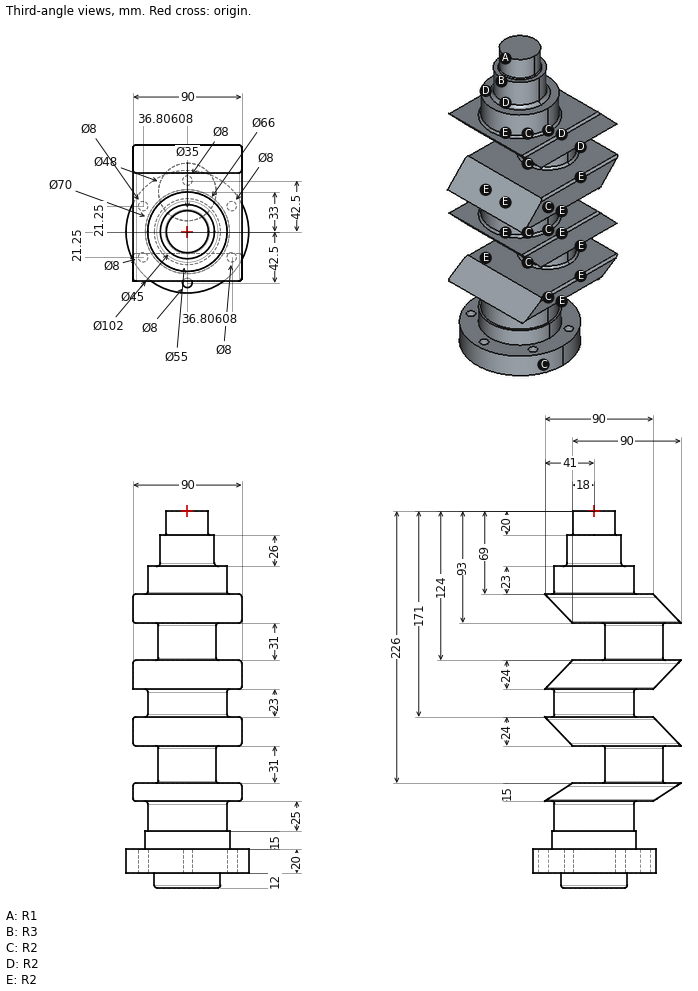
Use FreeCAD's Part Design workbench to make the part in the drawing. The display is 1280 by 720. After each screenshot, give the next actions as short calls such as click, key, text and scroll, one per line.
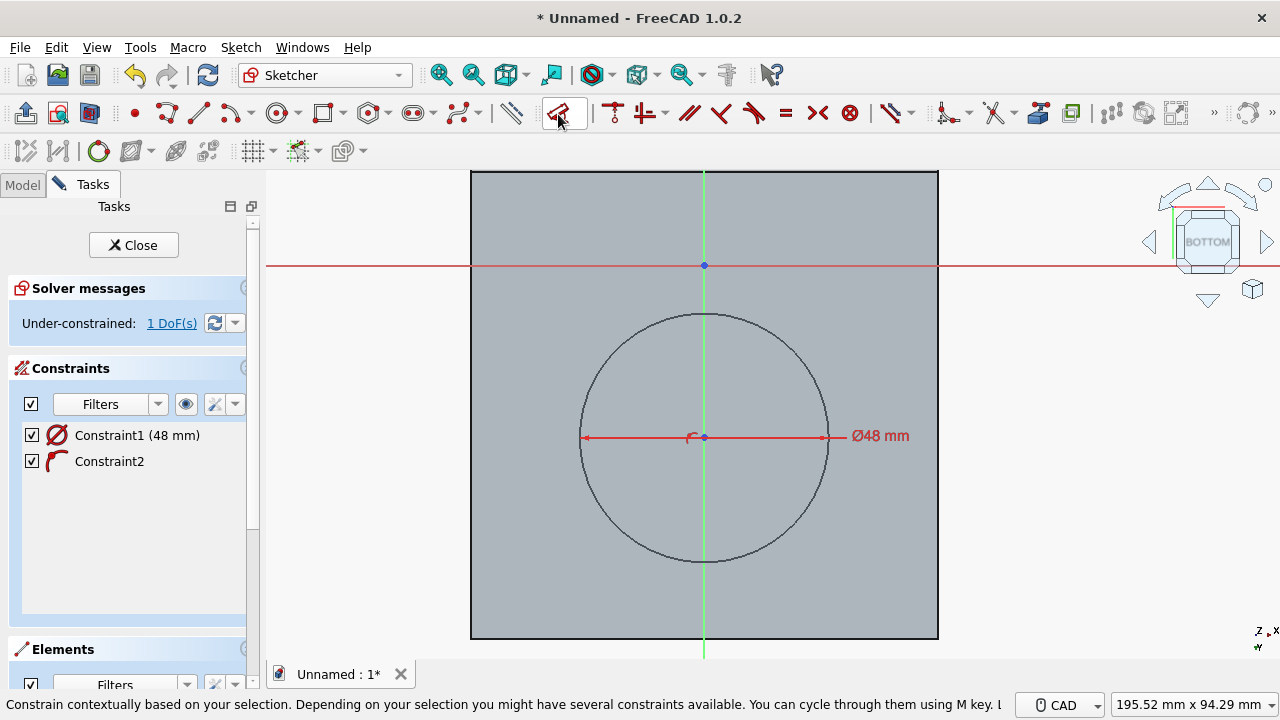
click(704, 438)
click(738, 352)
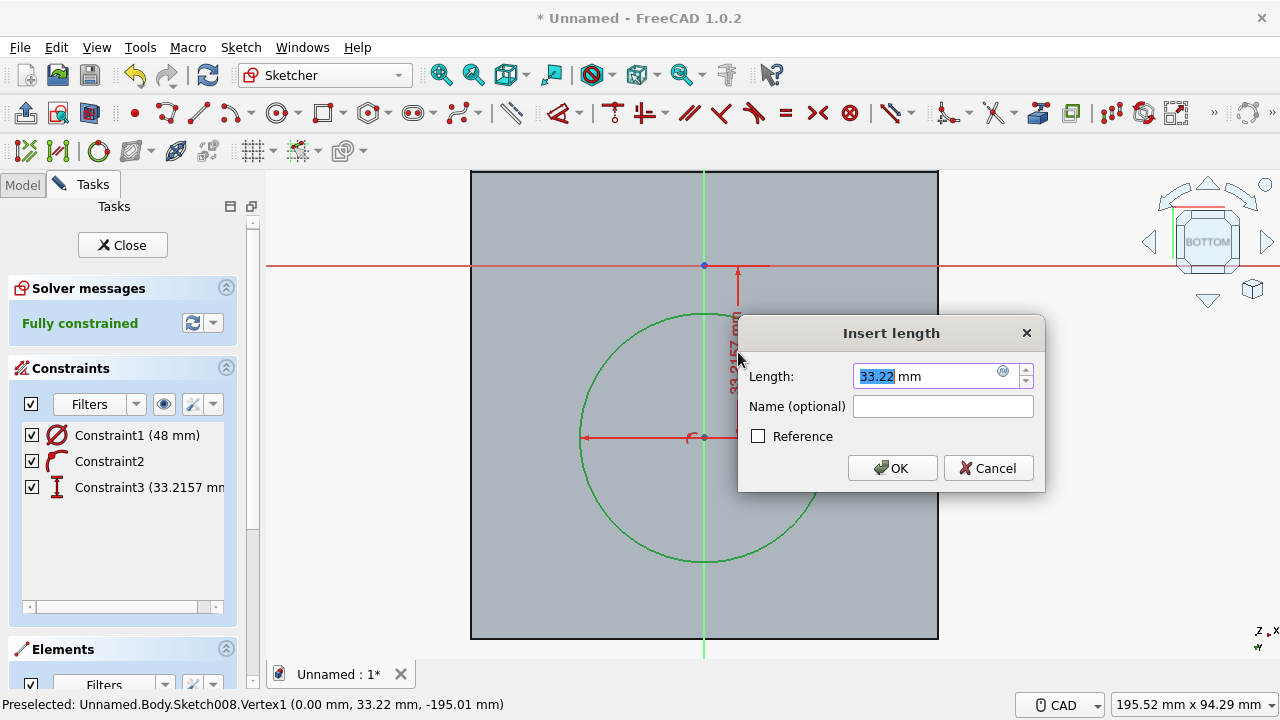
text(33)
key(Return)
key(Escape)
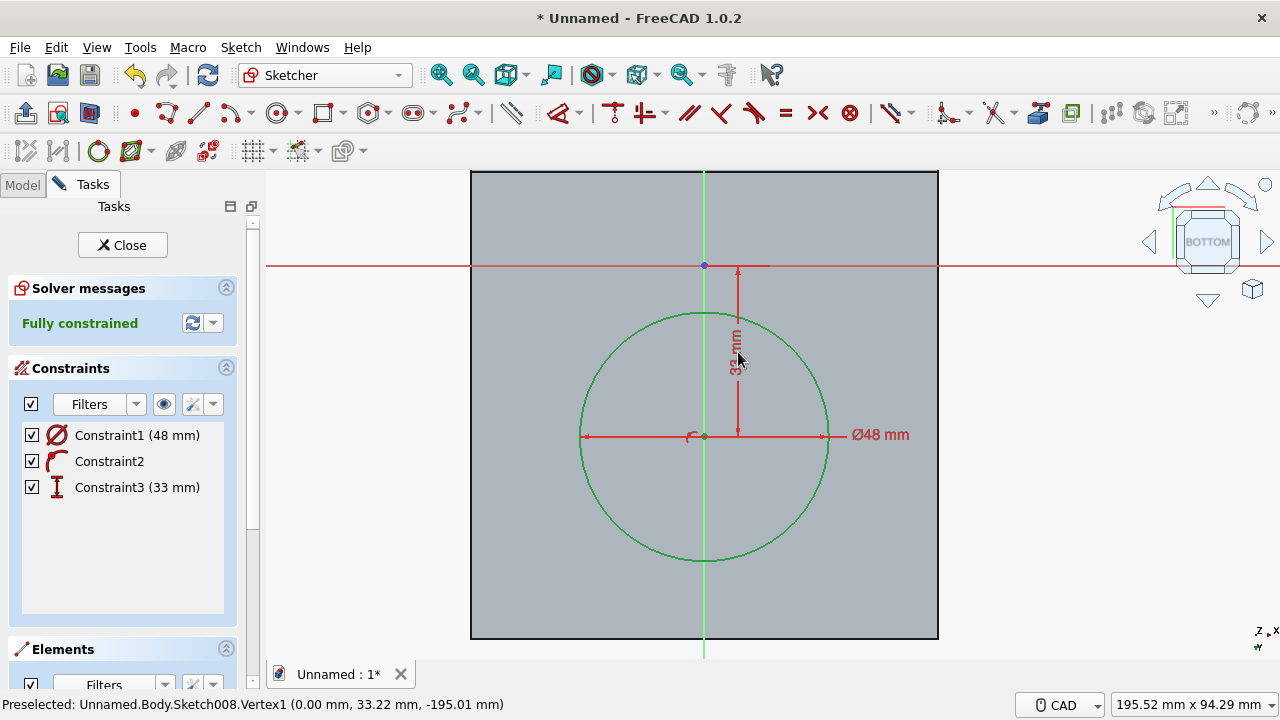
click(123, 245)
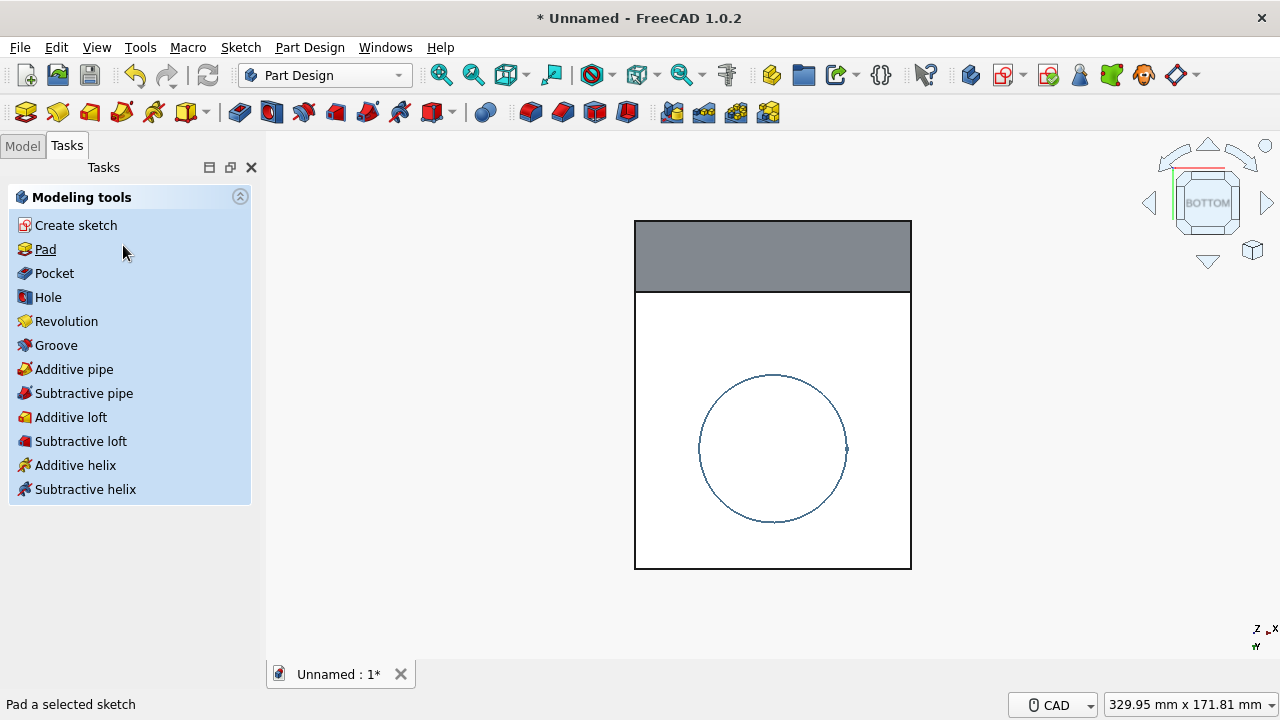
click(26, 112)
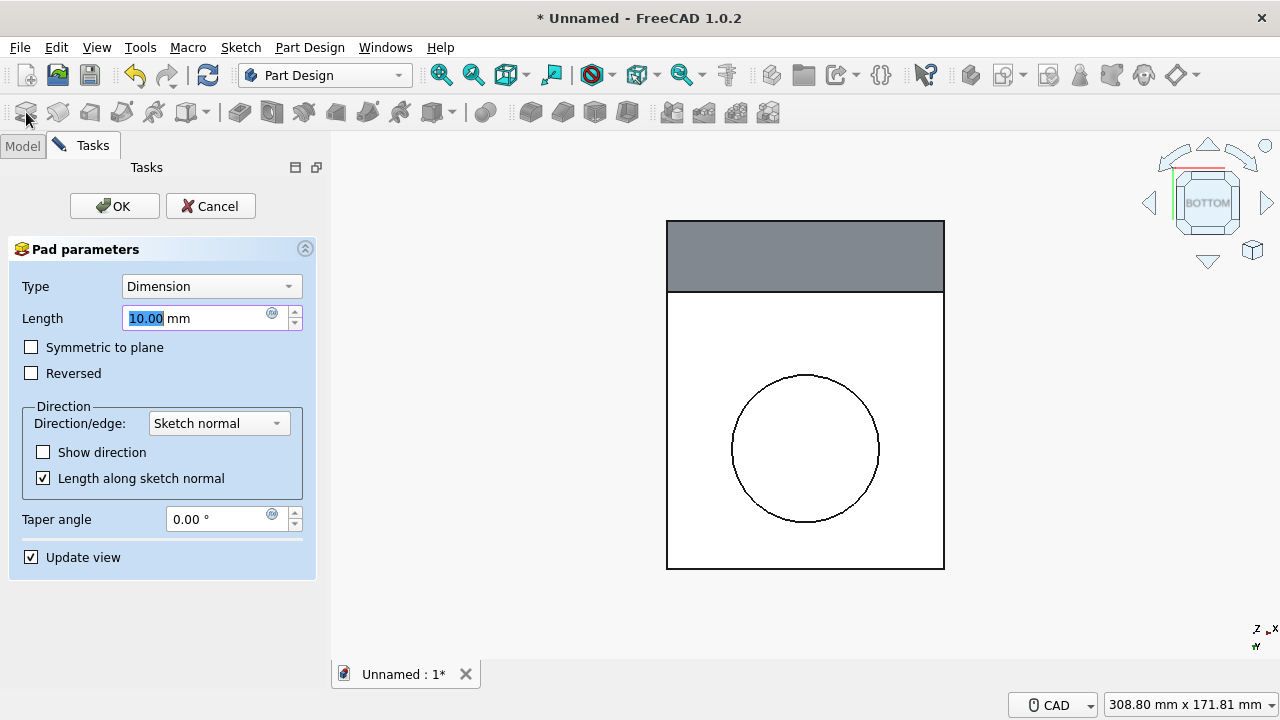
text(31)
key(Tab)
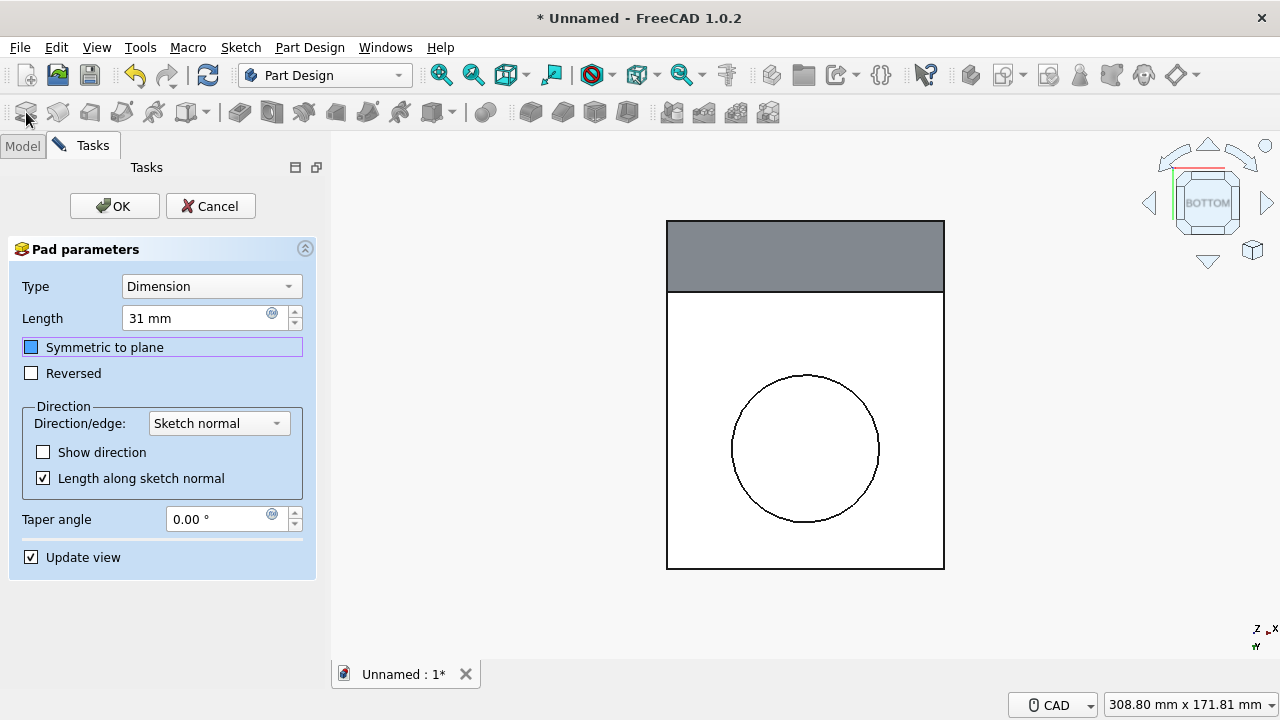
click(115, 206)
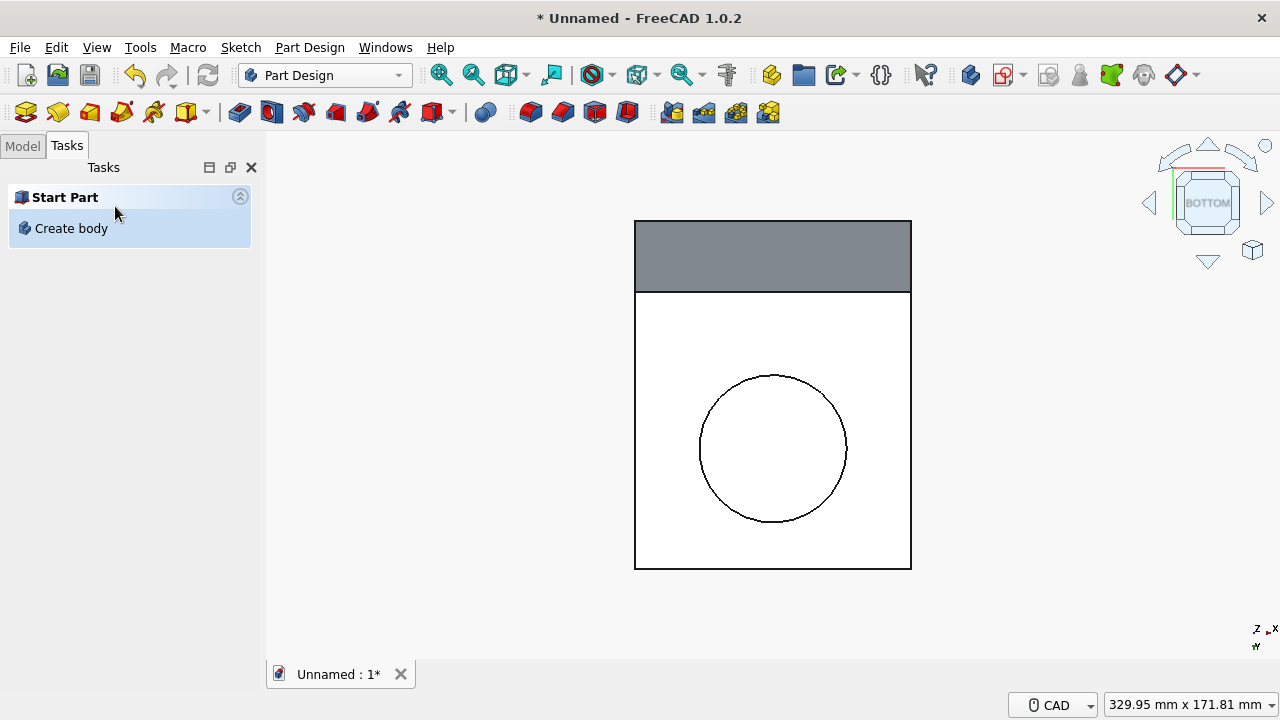
click(1004, 76)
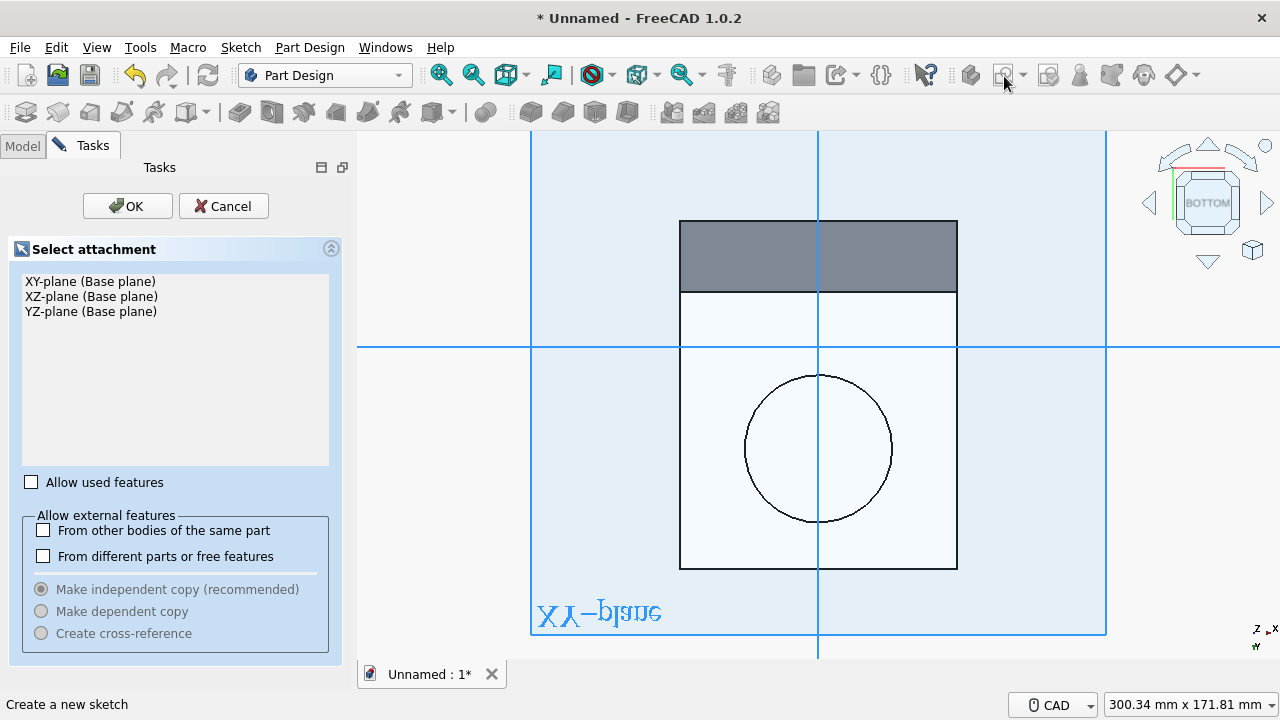
click(82, 312)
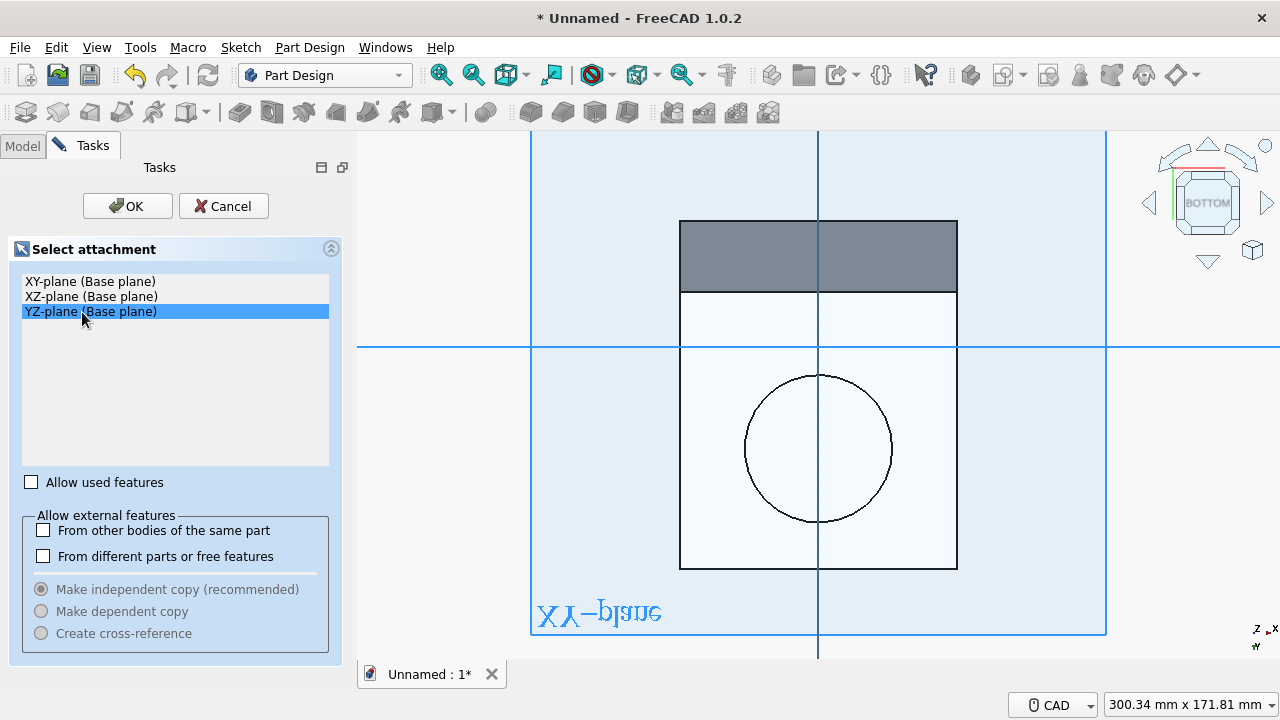
click(128, 206)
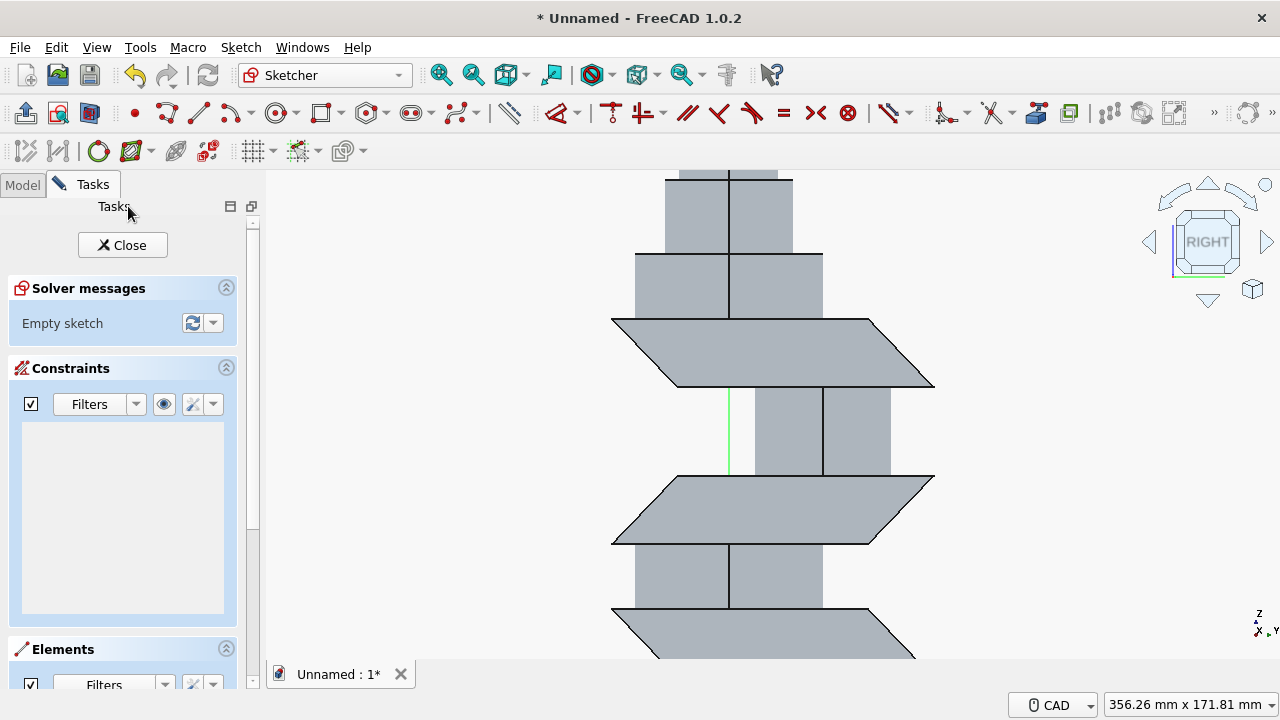
click(90, 114)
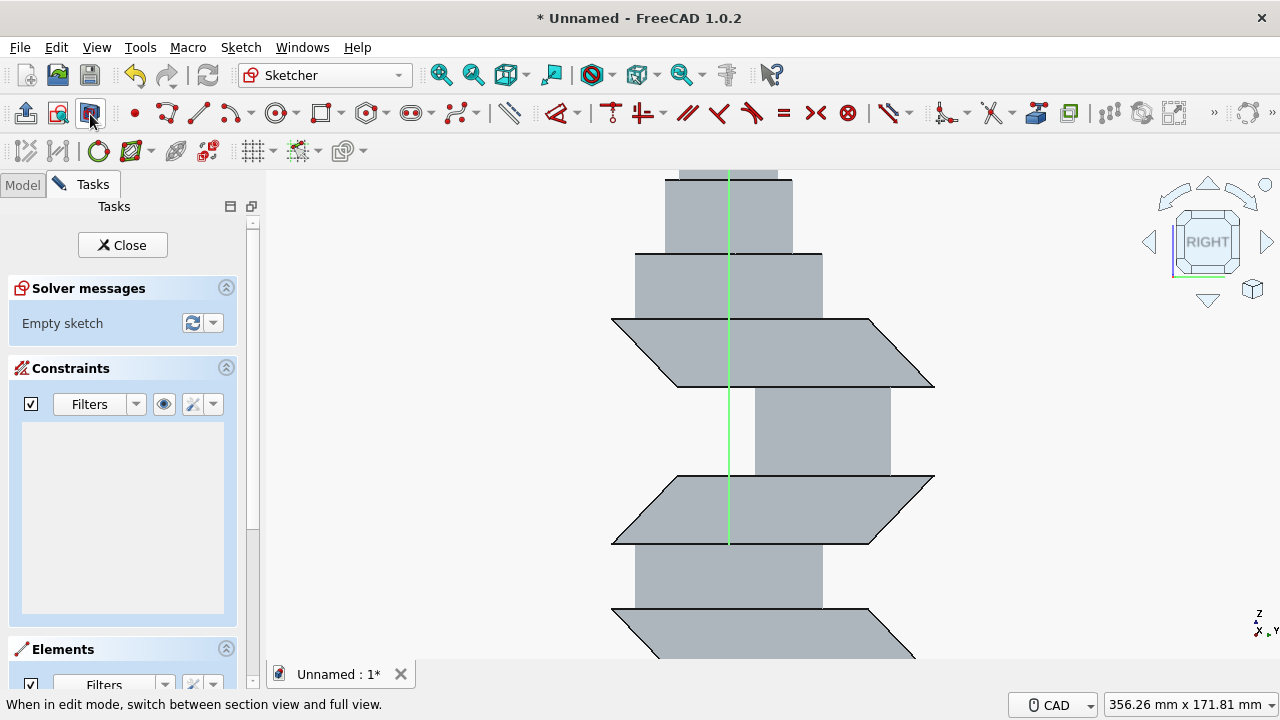
scroll(649, 373, down, 4)